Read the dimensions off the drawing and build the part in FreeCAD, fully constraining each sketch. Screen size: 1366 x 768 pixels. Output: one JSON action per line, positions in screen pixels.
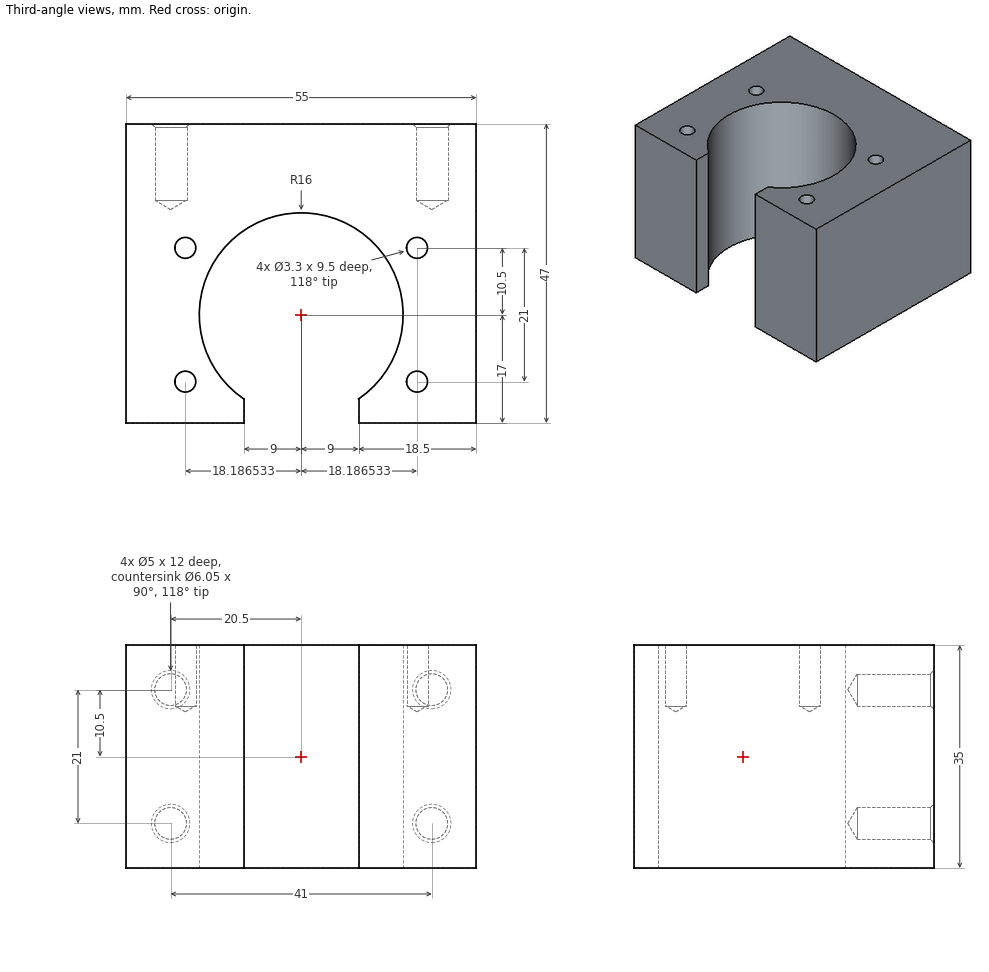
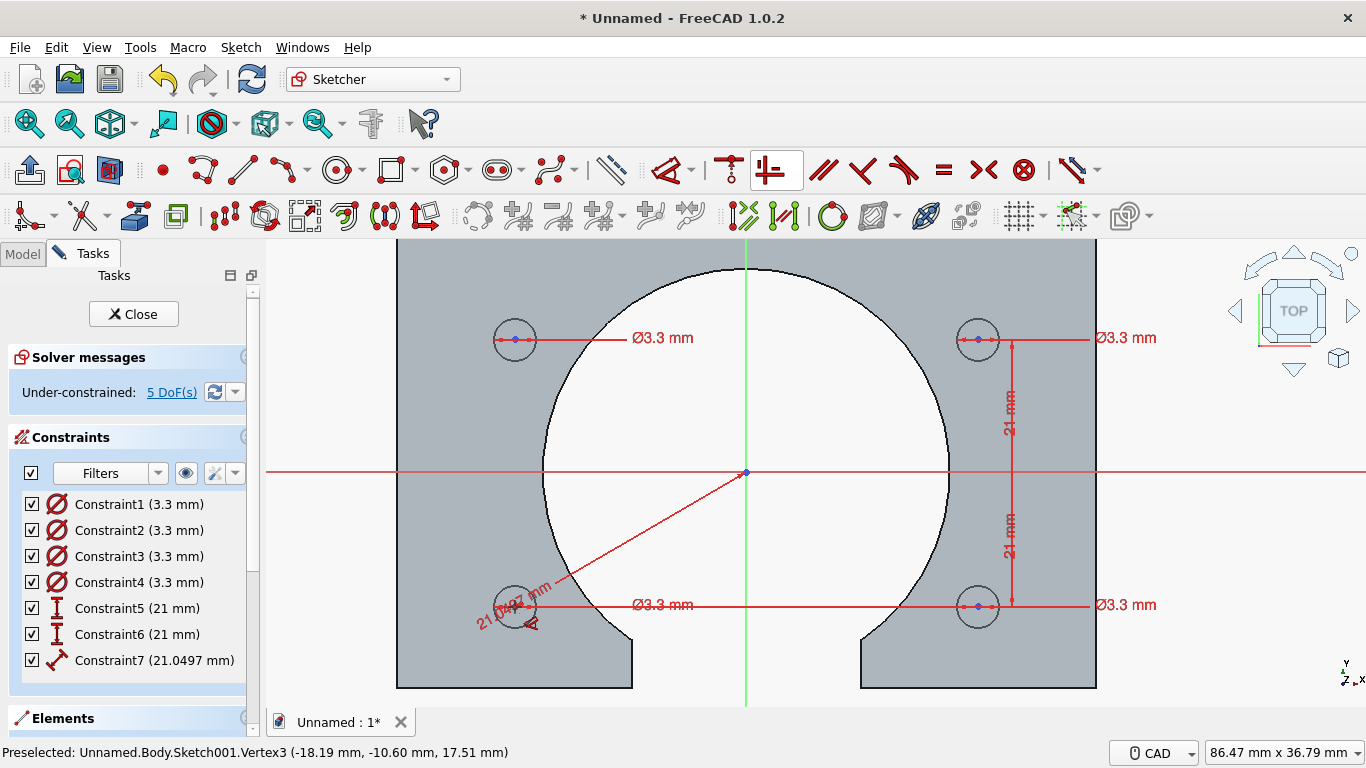
{"action": "left_click", "coordinate": [515, 340]}
{"action": "left_click", "coordinate": [481, 412]}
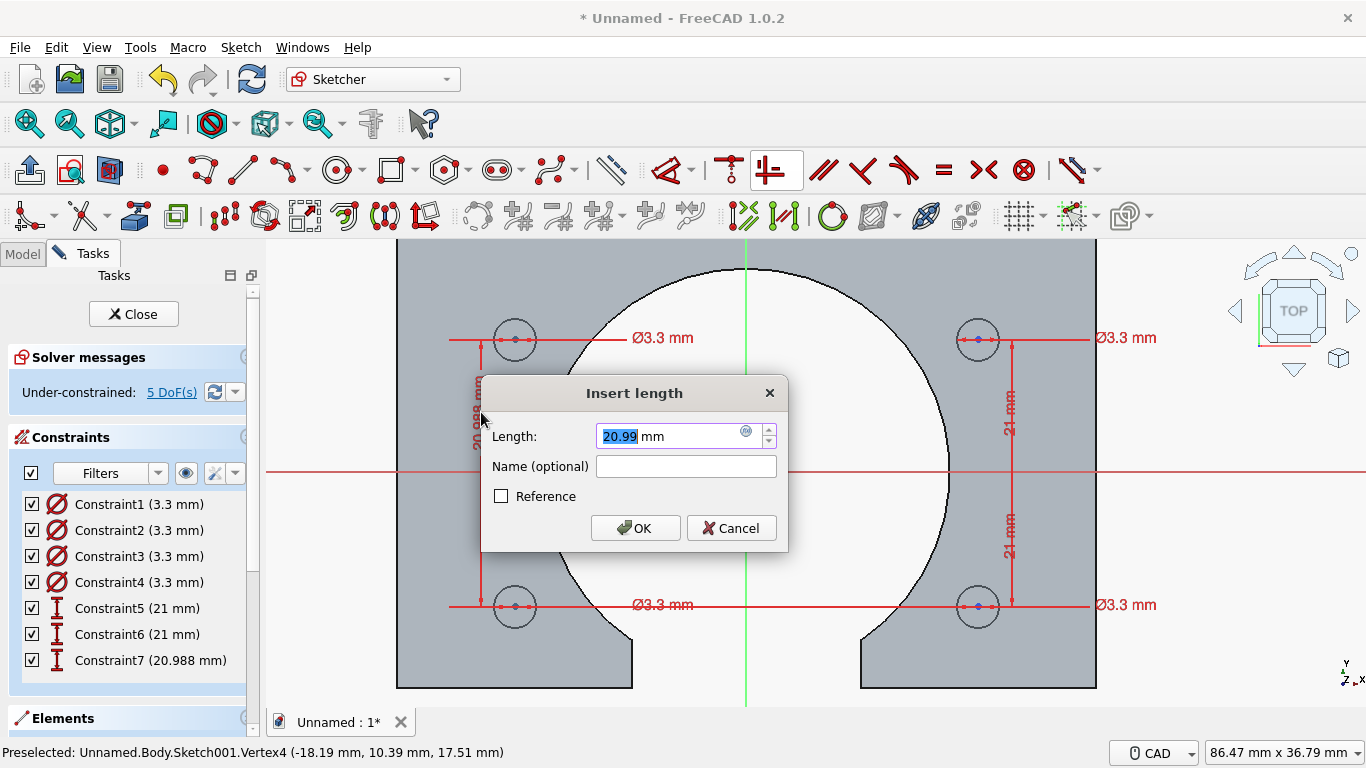
{"action": "type", "text": "21"}
{"action": "key", "text": "Return"}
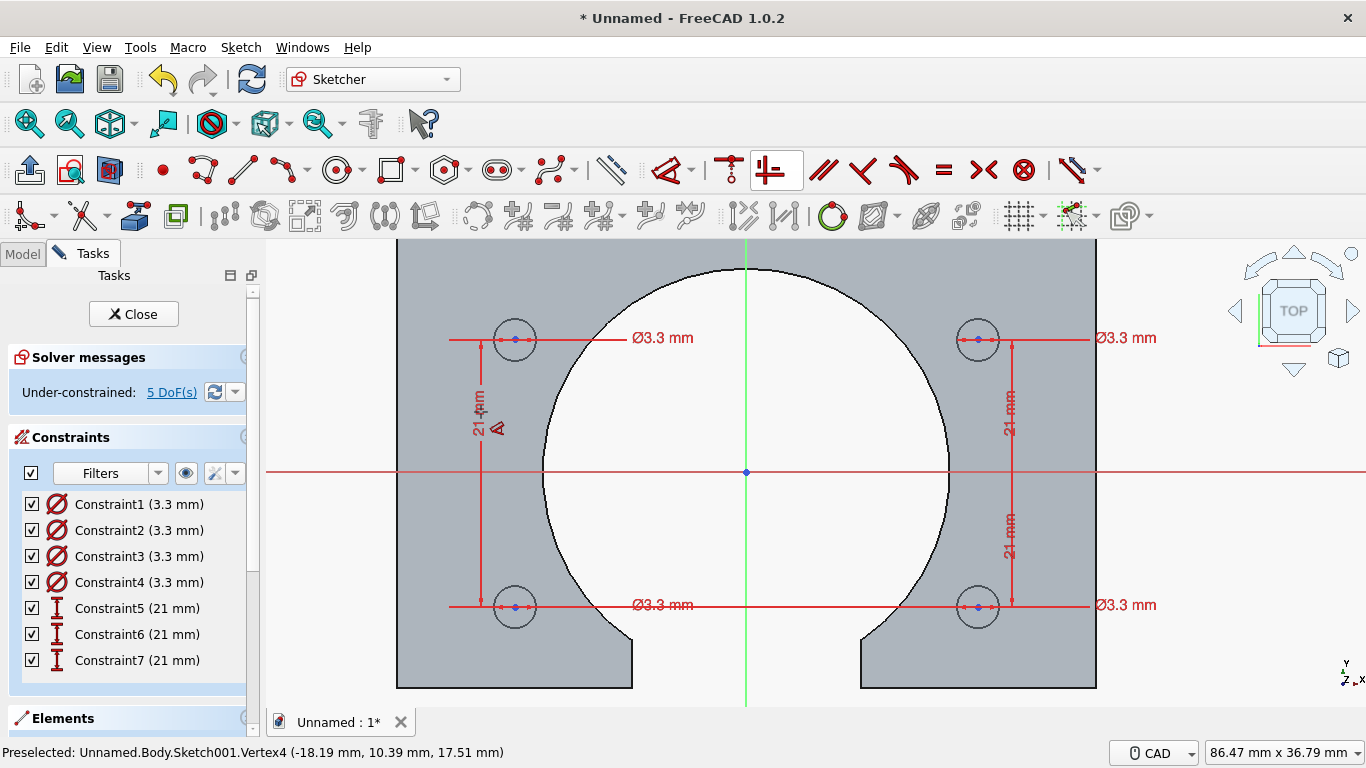
{"action": "left_click", "coordinate": [978, 340]}
{"action": "left_click", "coordinate": [1012, 376]}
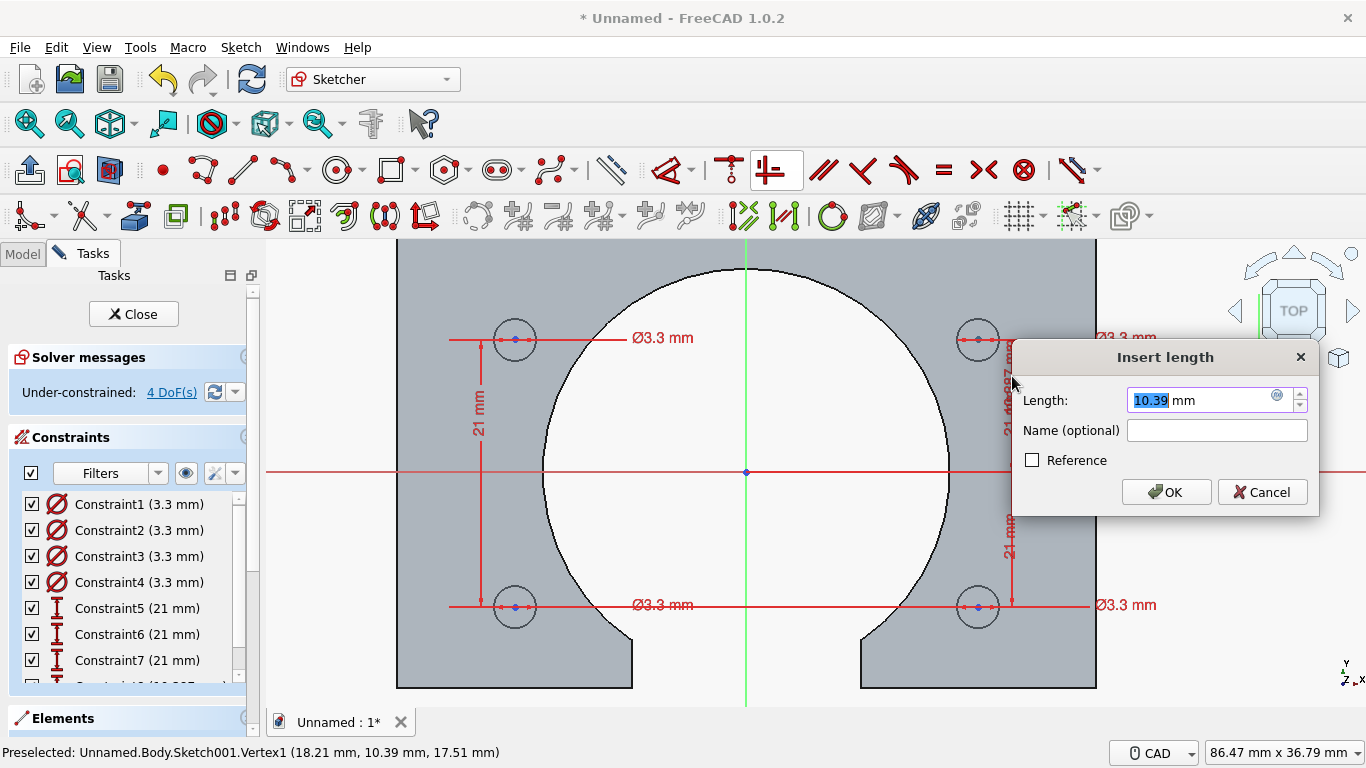
{"action": "type", "text": "10.5"}
{"action": "key", "text": "Return"}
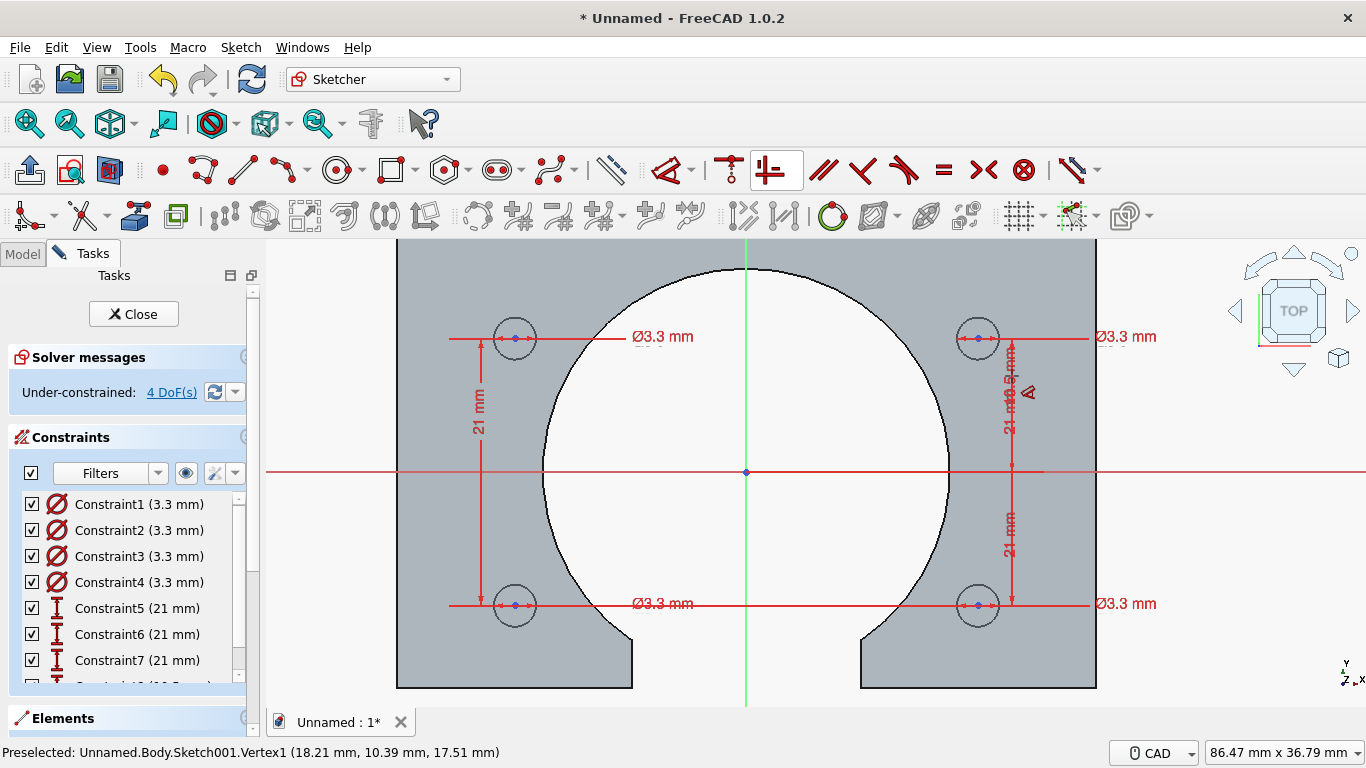
{"action": "left_click", "coordinate": [978, 339]}
{"action": "left_click", "coordinate": [862, 305]}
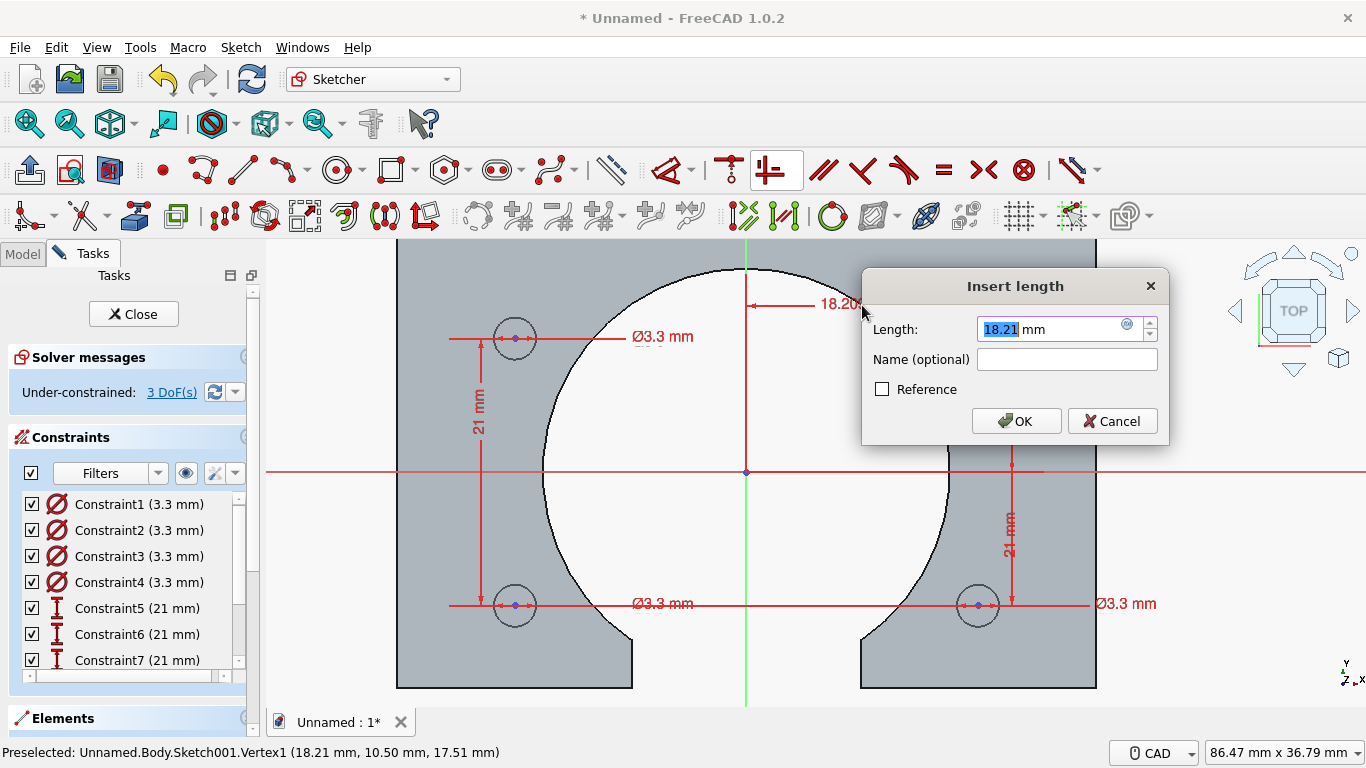
{"action": "type", "text": "18.186533"}
{"action": "key", "text": "Return"}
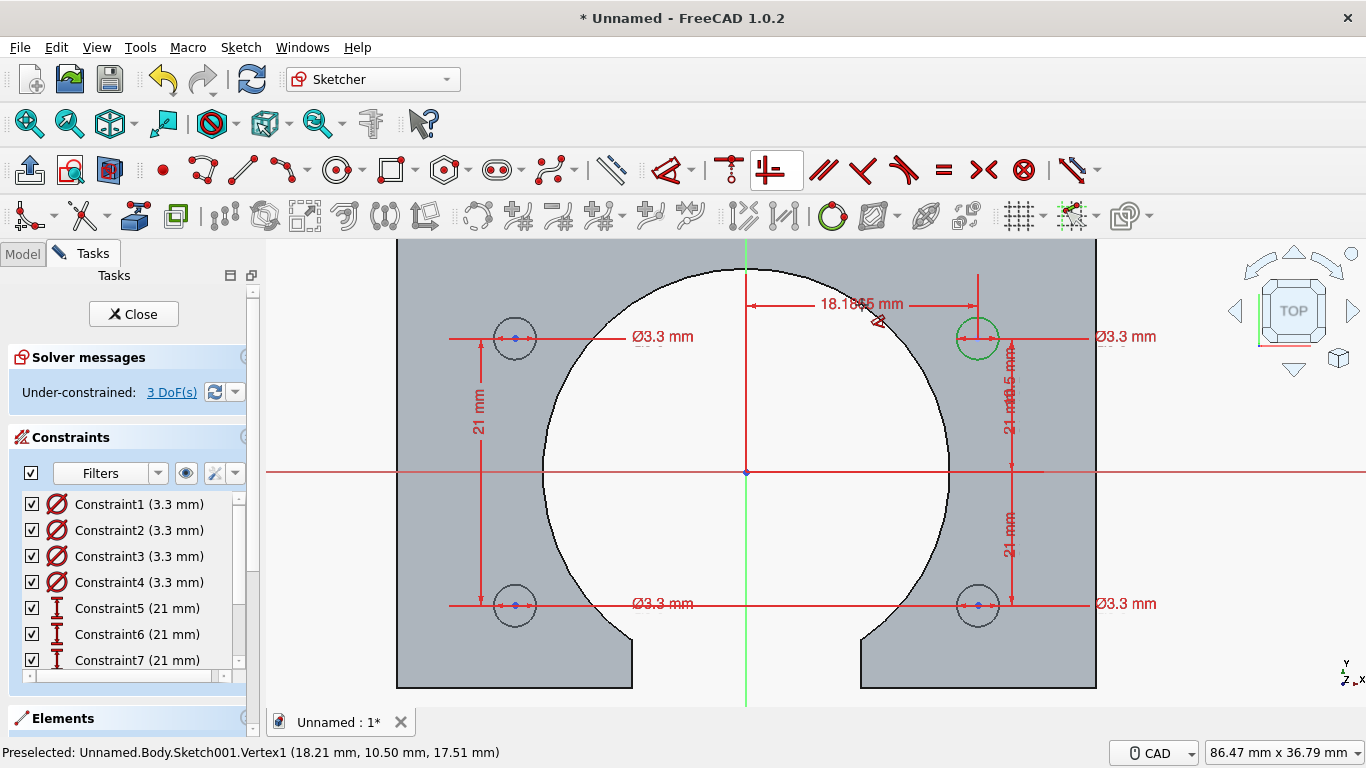
{"action": "left_click", "coordinate": [978, 606]}
{"action": "left_click", "coordinate": [862, 640]}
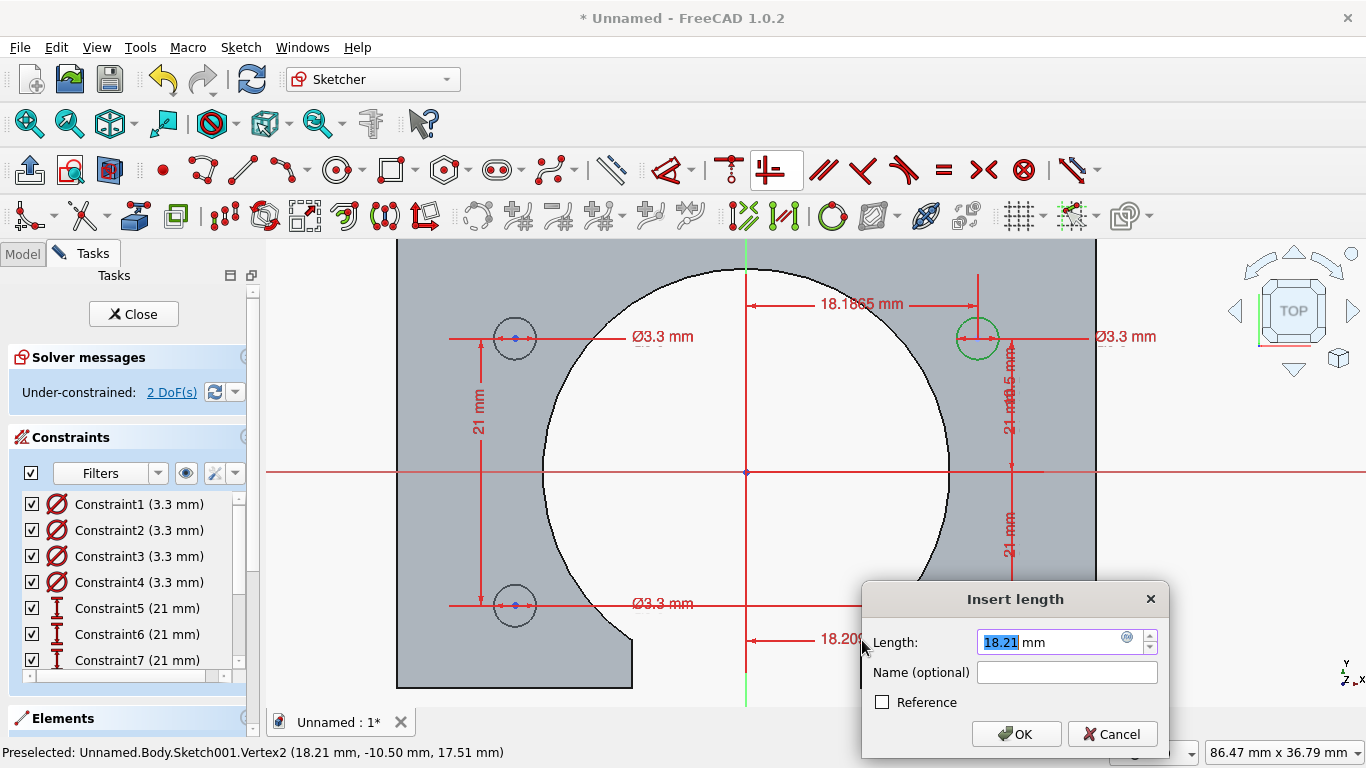
{"action": "type", "text": "18.186533"}
{"action": "key", "text": "Return"}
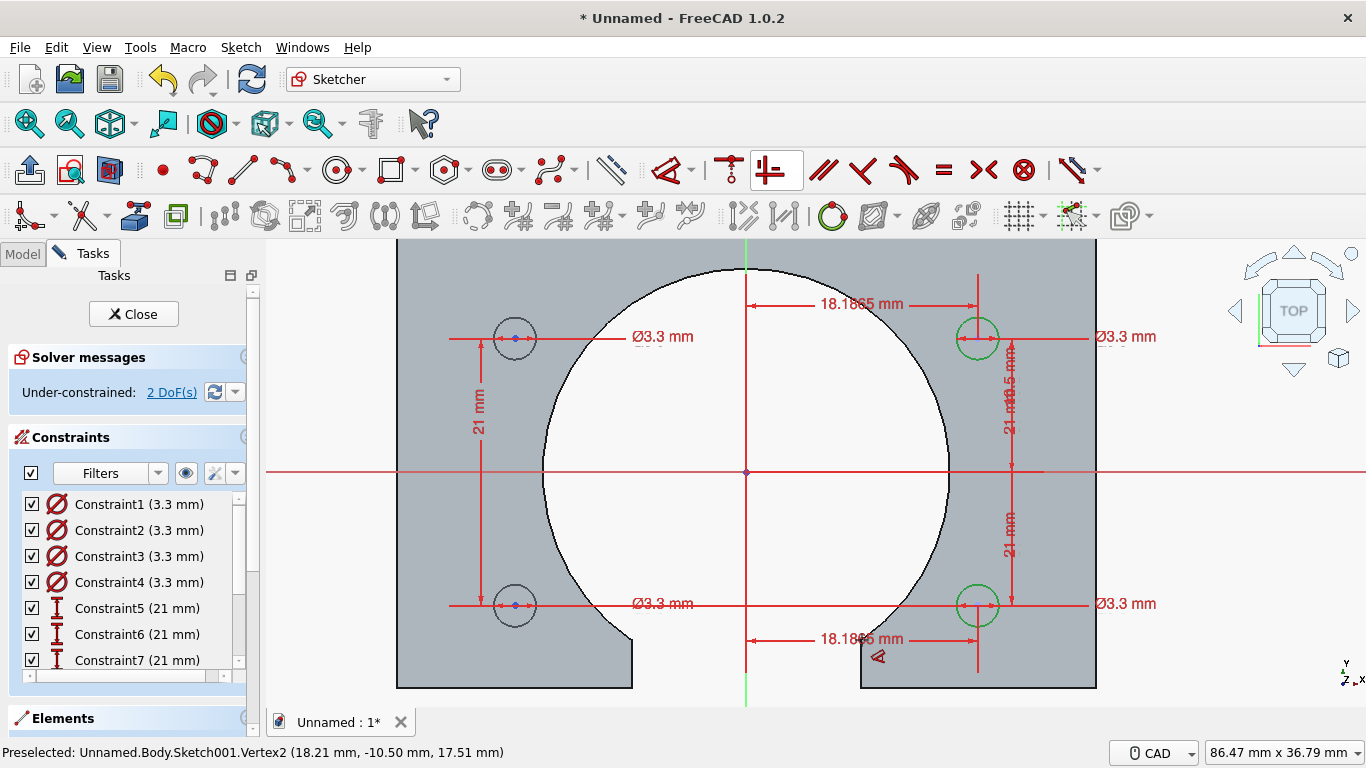
{"action": "left_click", "coordinate": [515, 606]}
{"action": "left_click", "coordinate": [631, 640]}